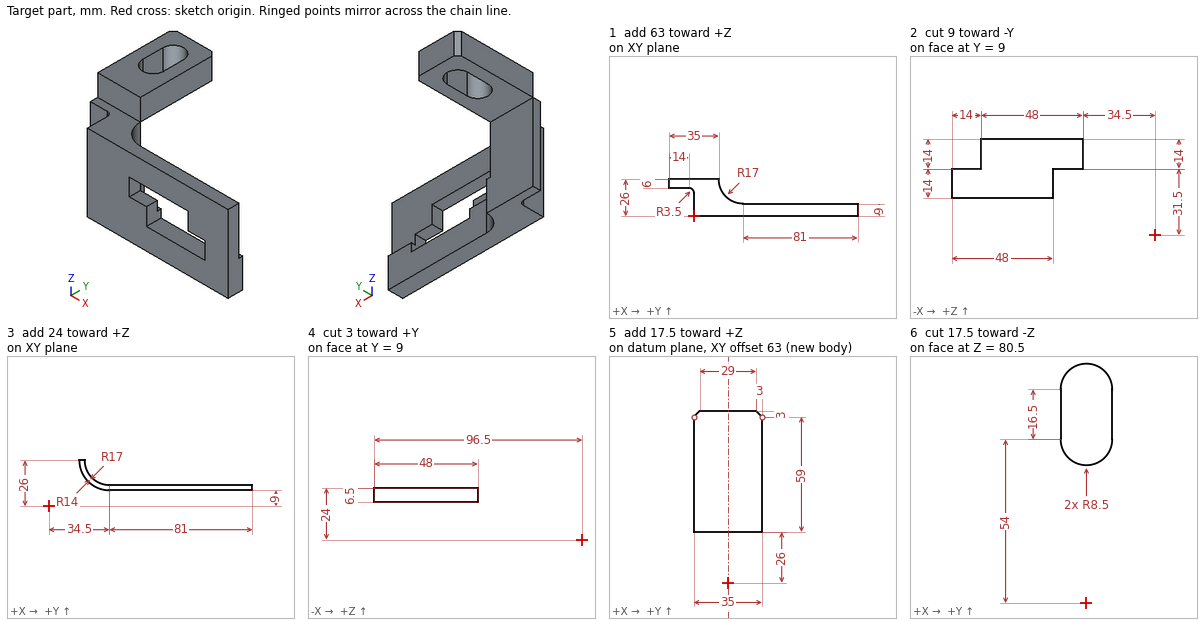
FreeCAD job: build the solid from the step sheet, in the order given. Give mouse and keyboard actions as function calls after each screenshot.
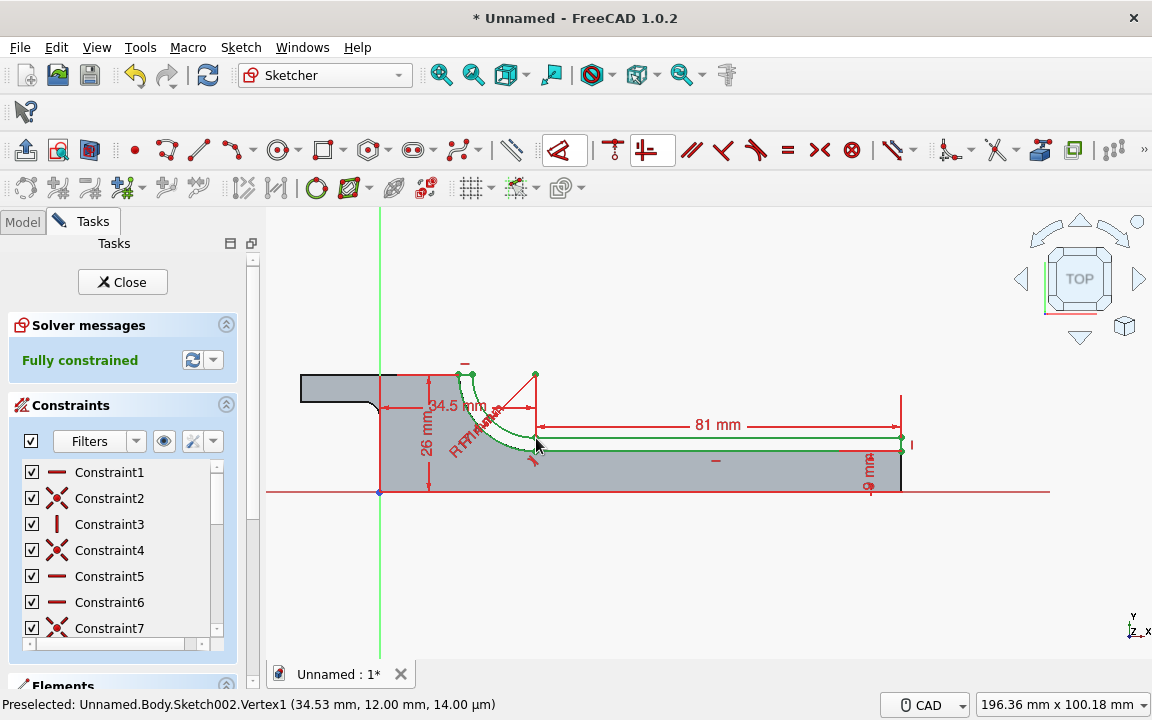
click(123, 282)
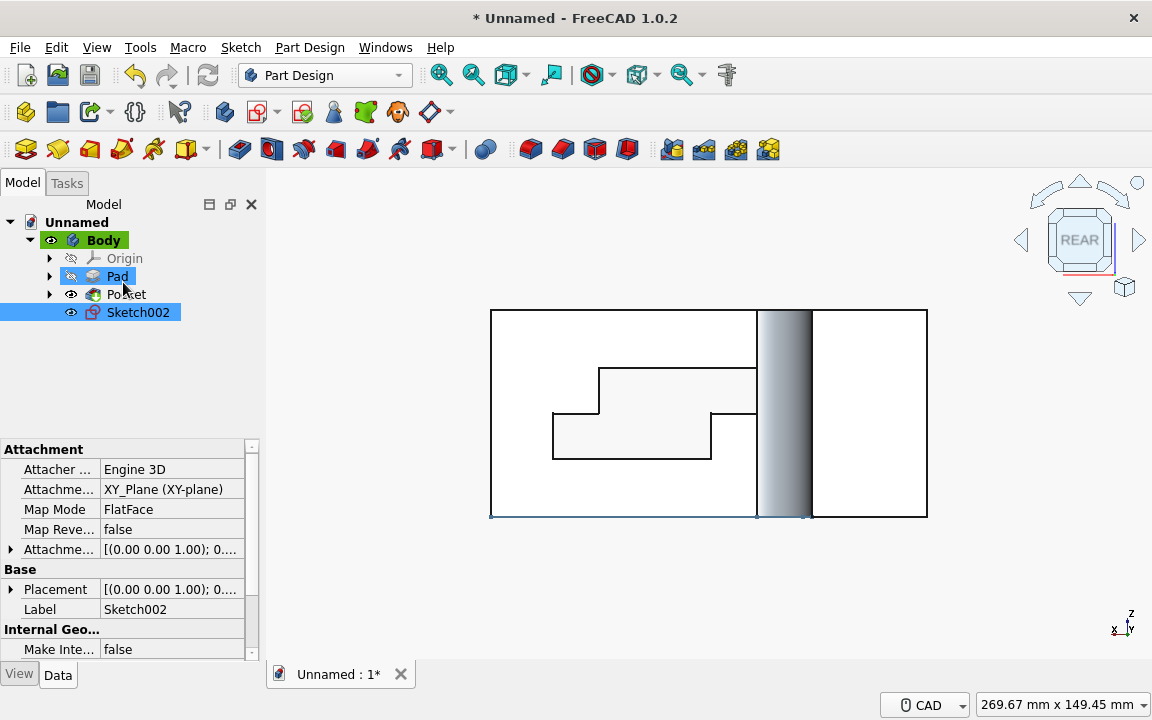
click(26, 150)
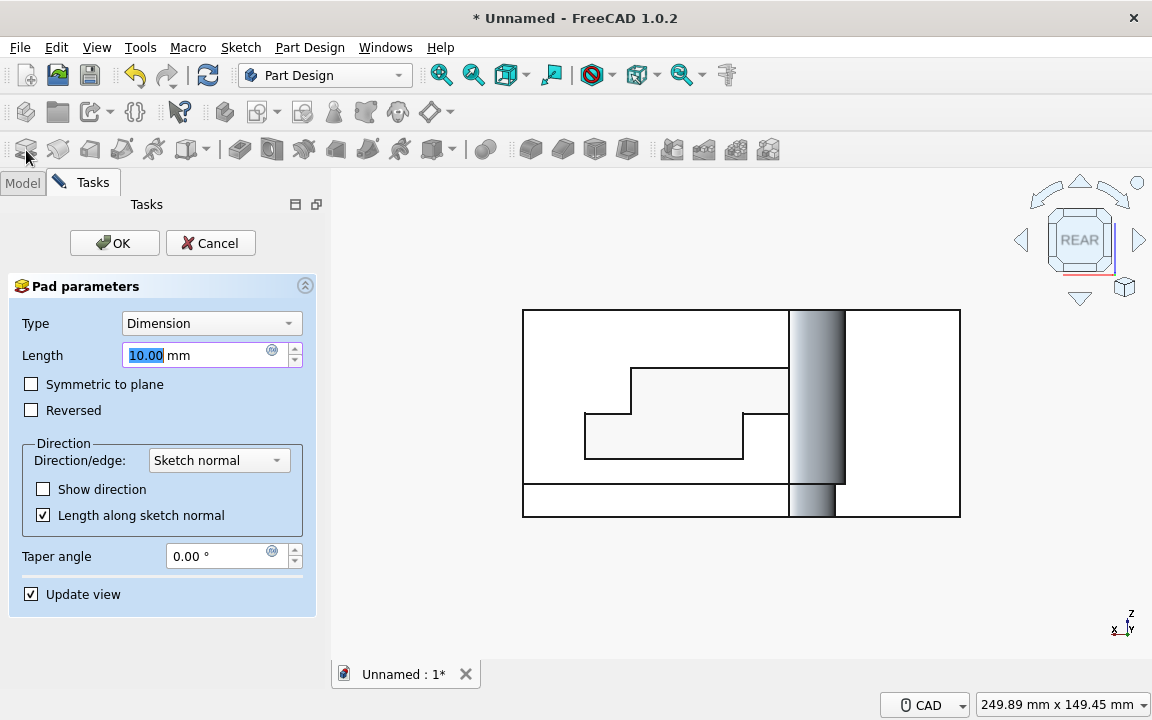
text(24)
key(Tab)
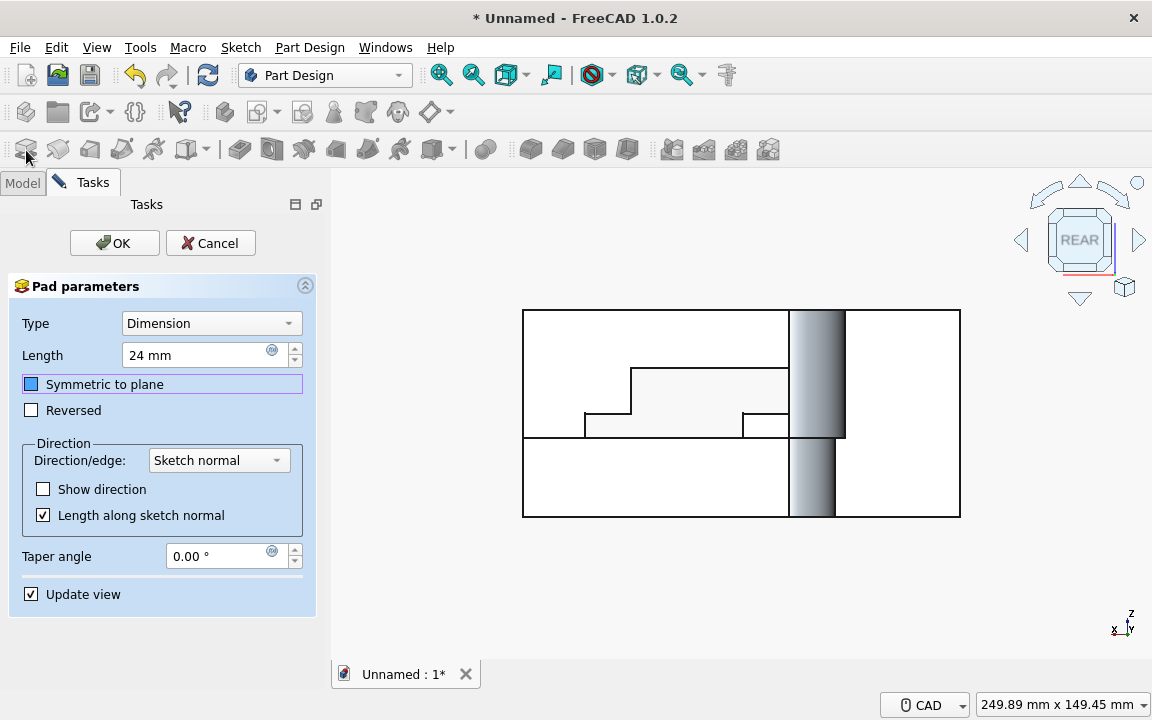
click(115, 243)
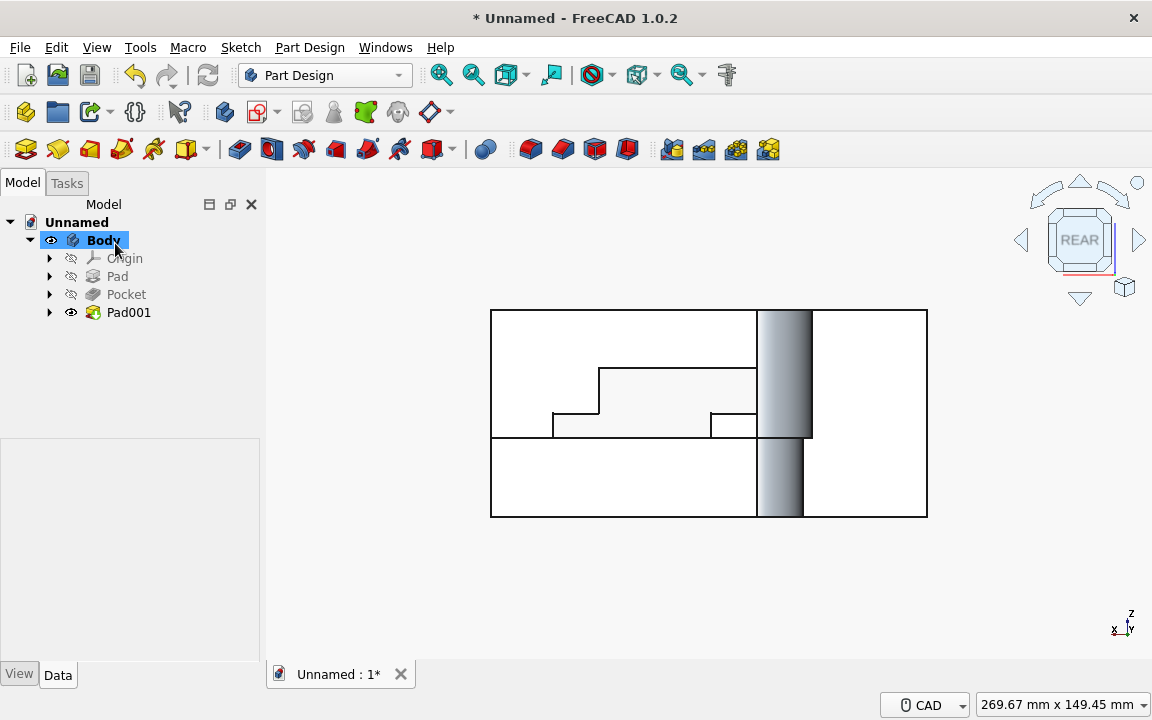
click(548, 355)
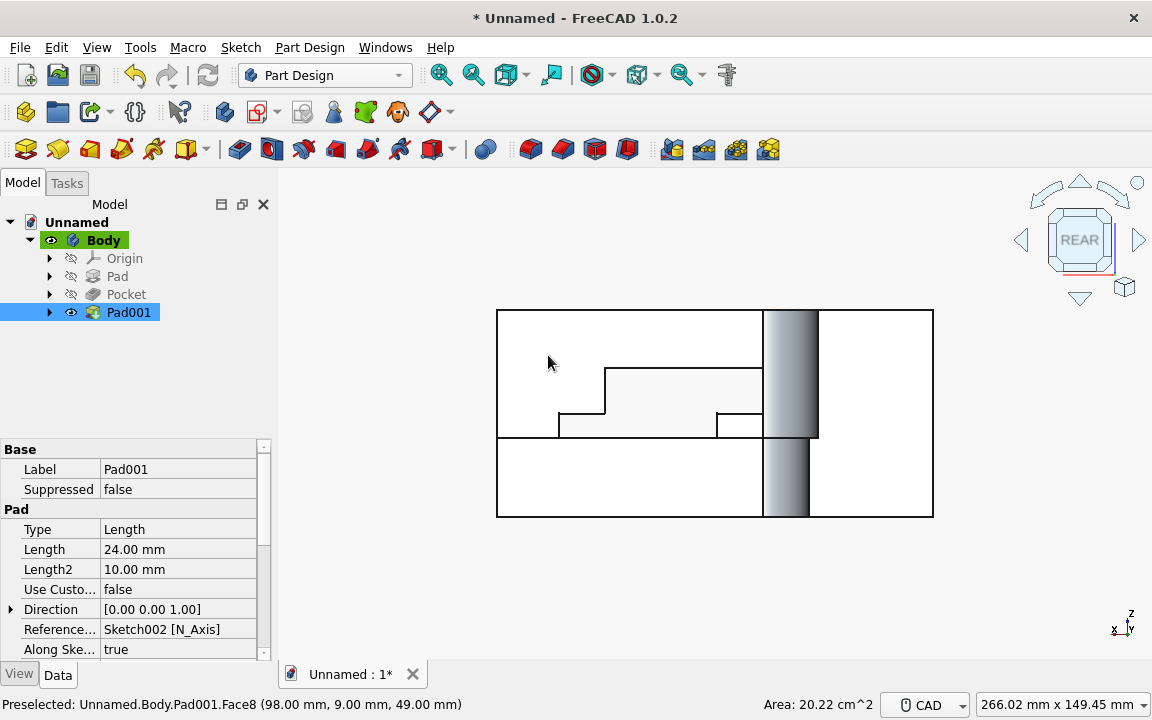
click(258, 112)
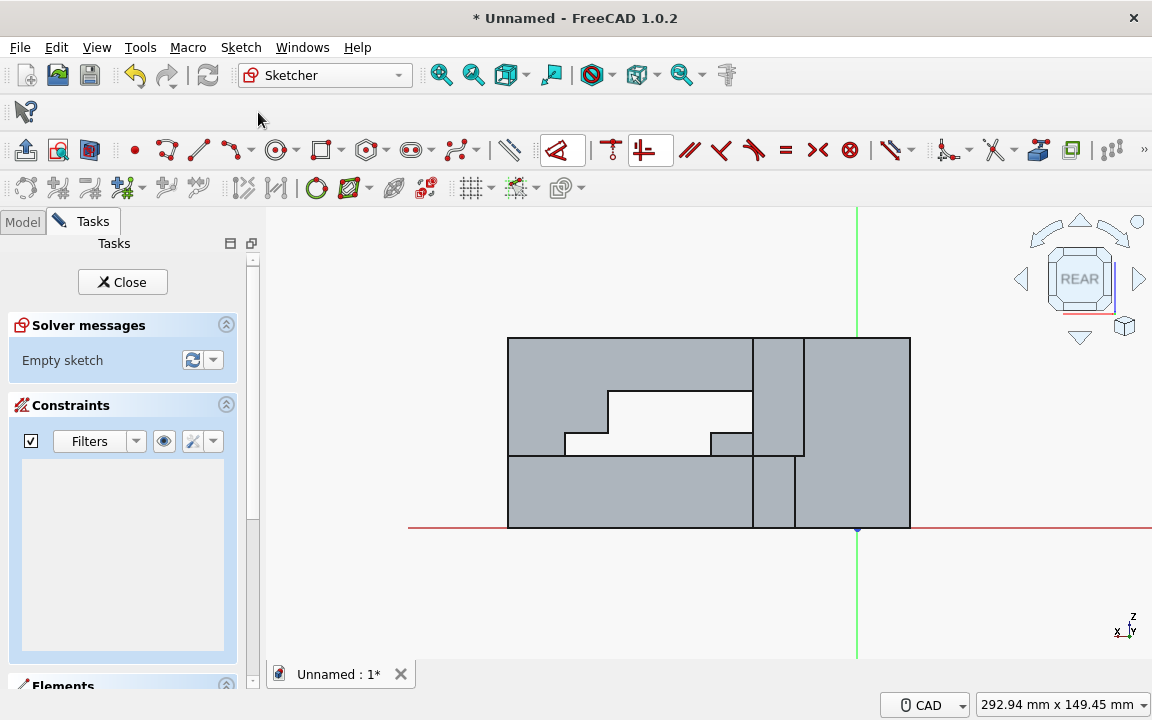
scroll(797, 564, up, 3)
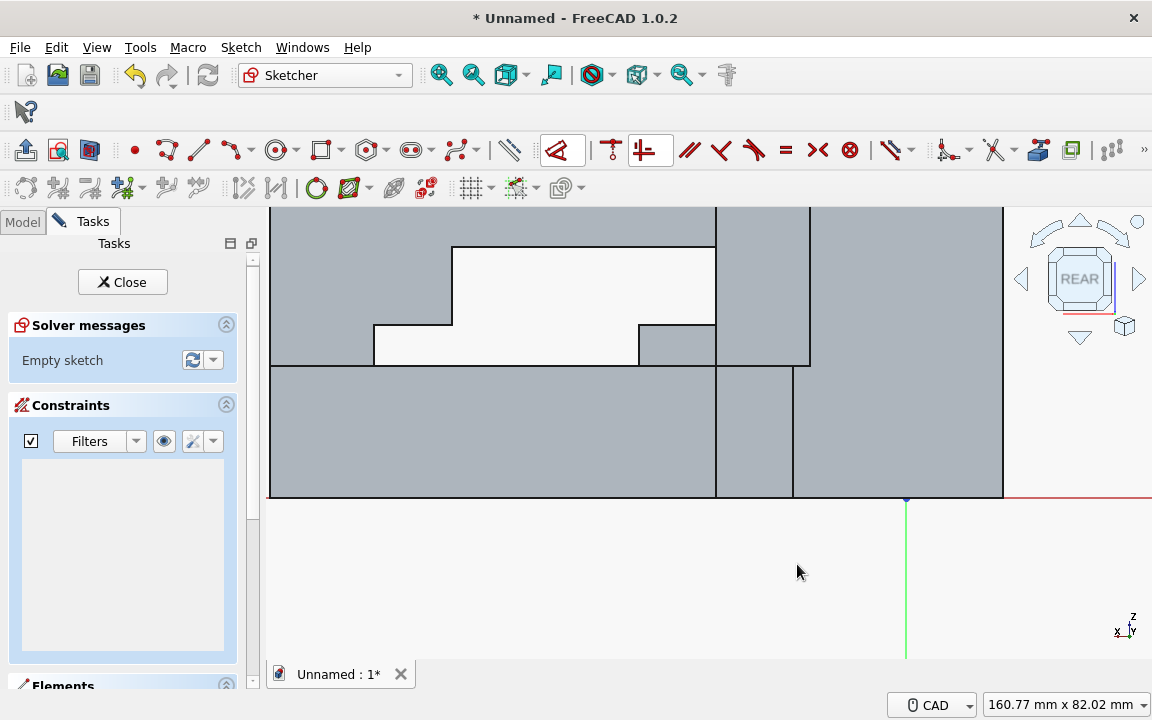
key(g)
key(r)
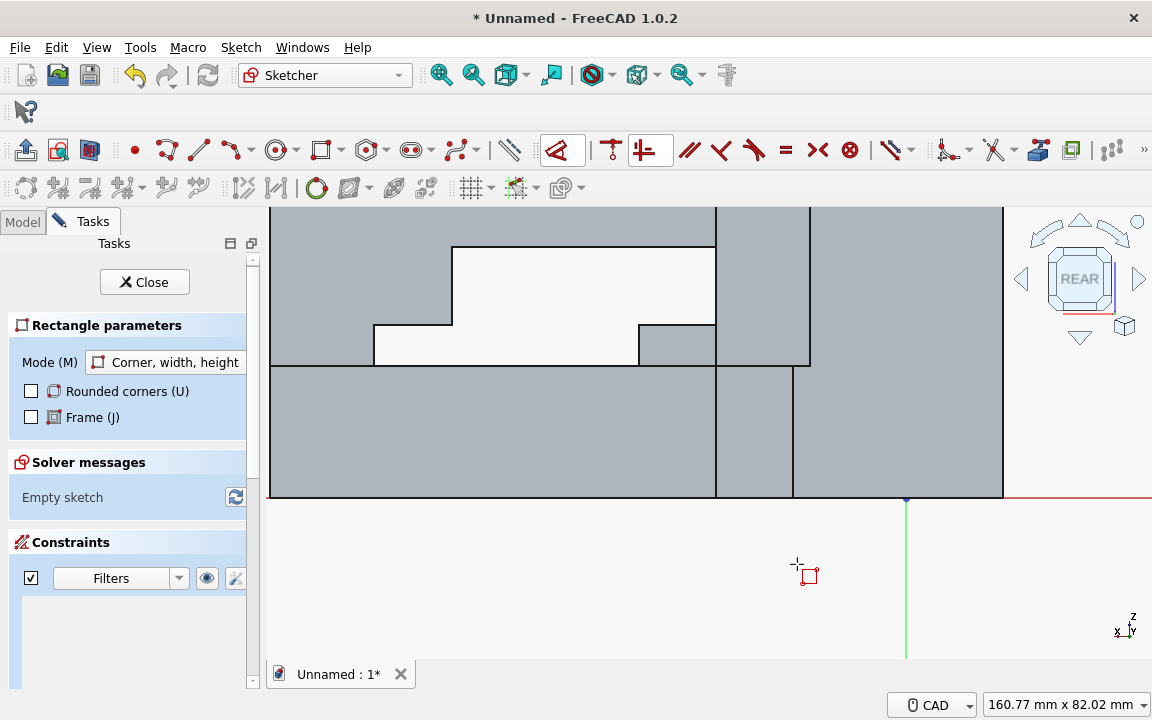
click(374, 366)
move(639, 402)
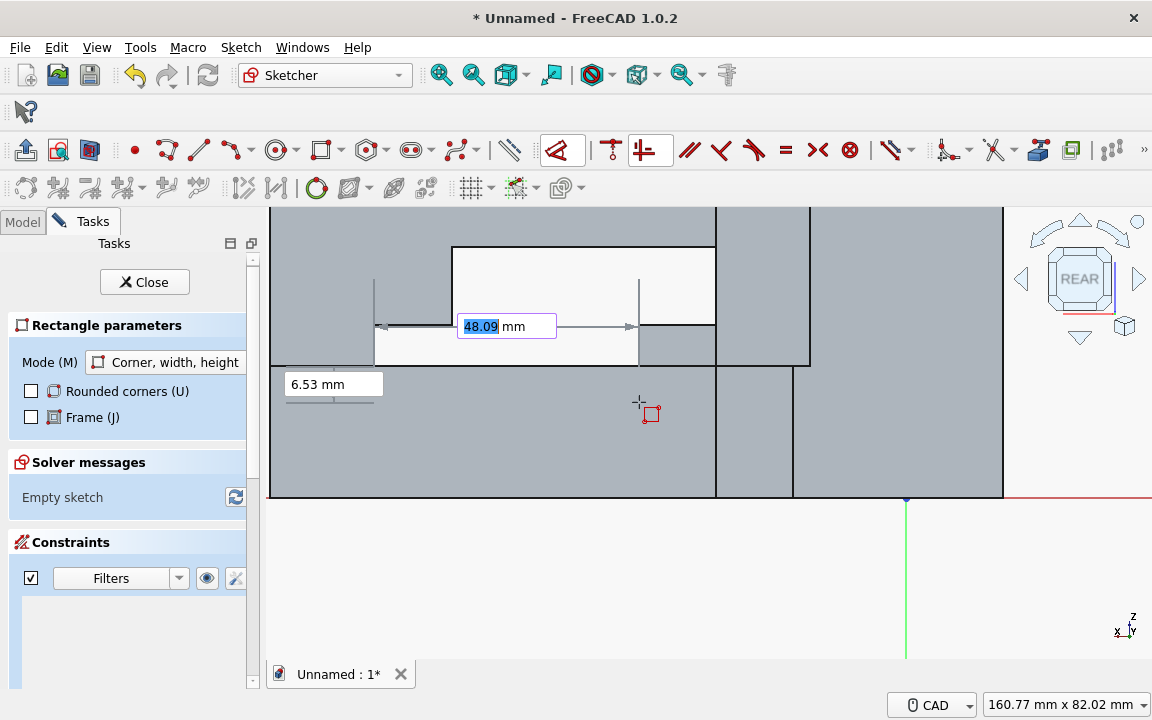
text(48)
key(Tab)
text(6.5)
key(Return)
key(Escape)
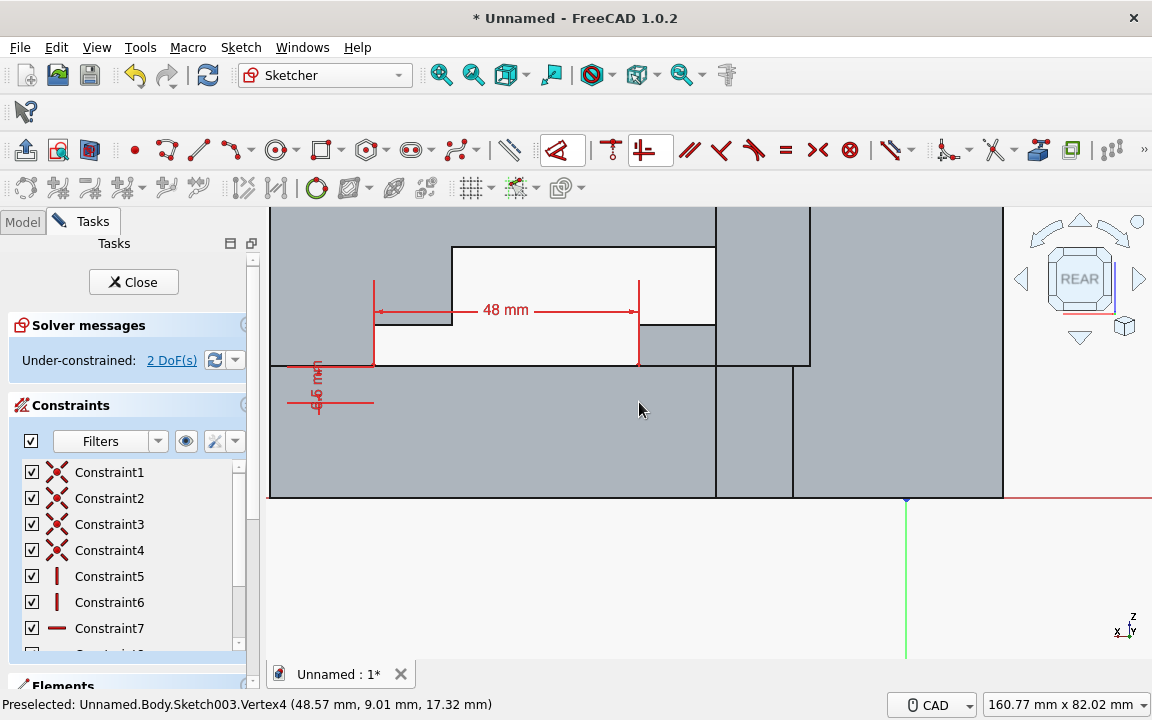
click(374, 367)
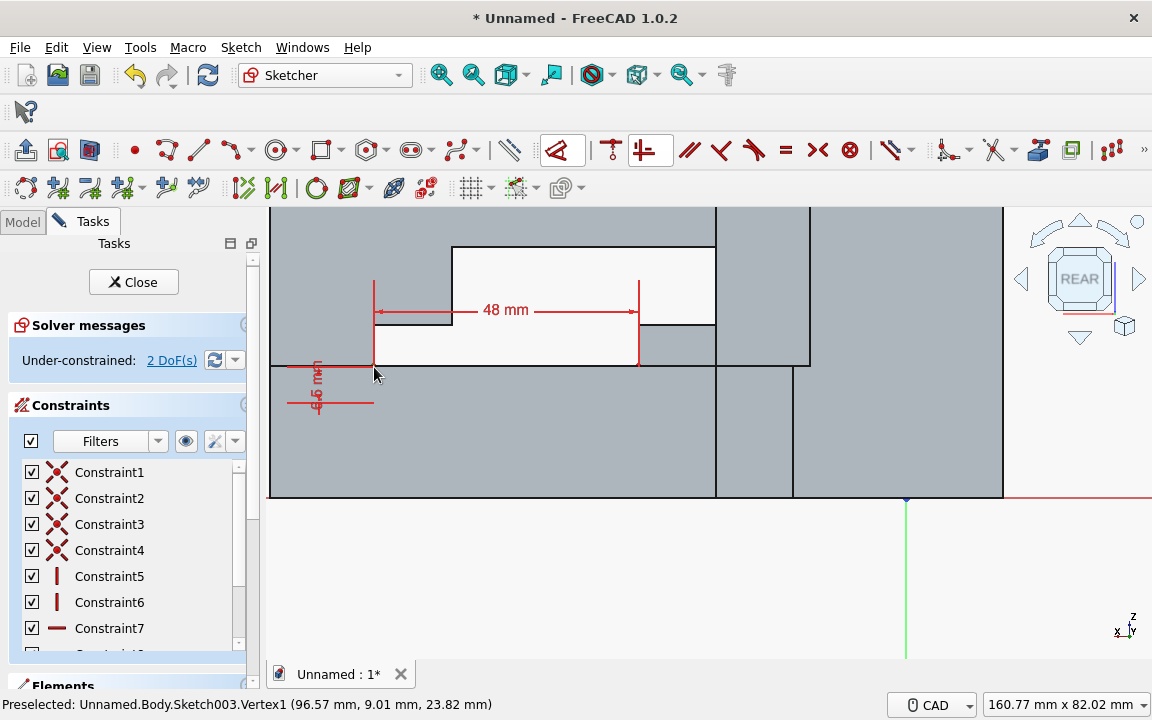
key(i)